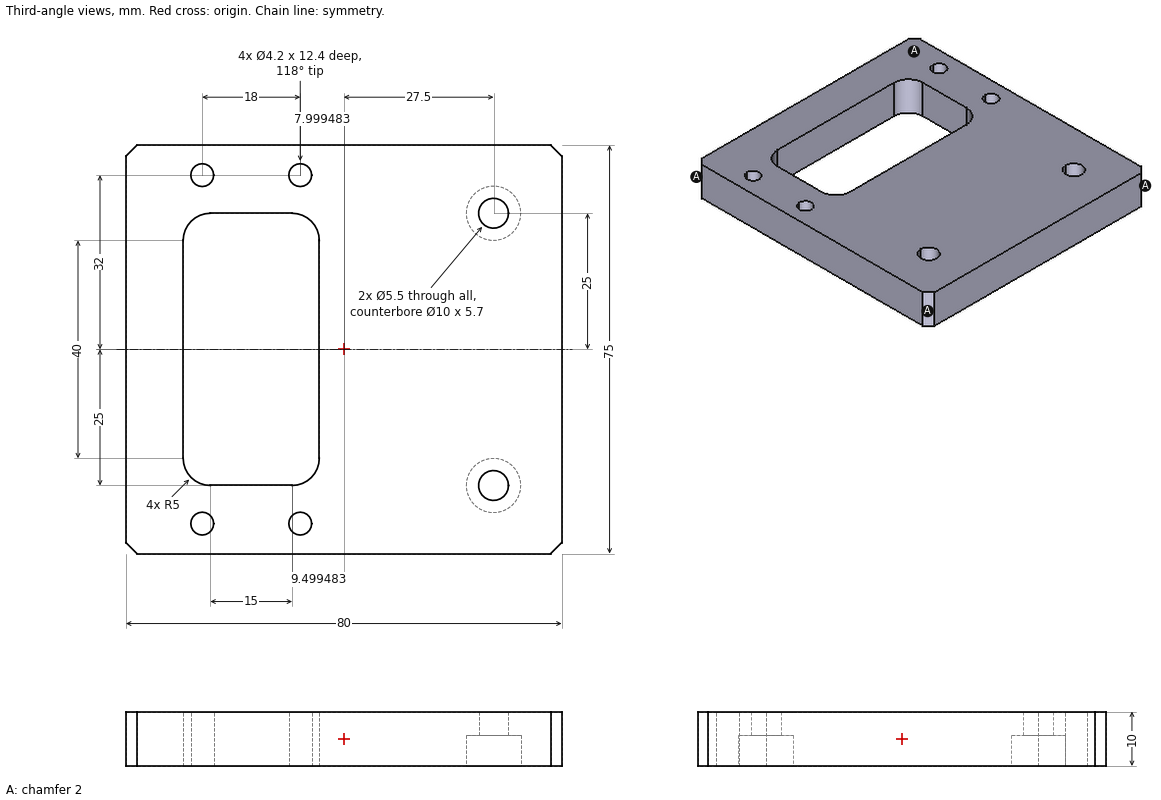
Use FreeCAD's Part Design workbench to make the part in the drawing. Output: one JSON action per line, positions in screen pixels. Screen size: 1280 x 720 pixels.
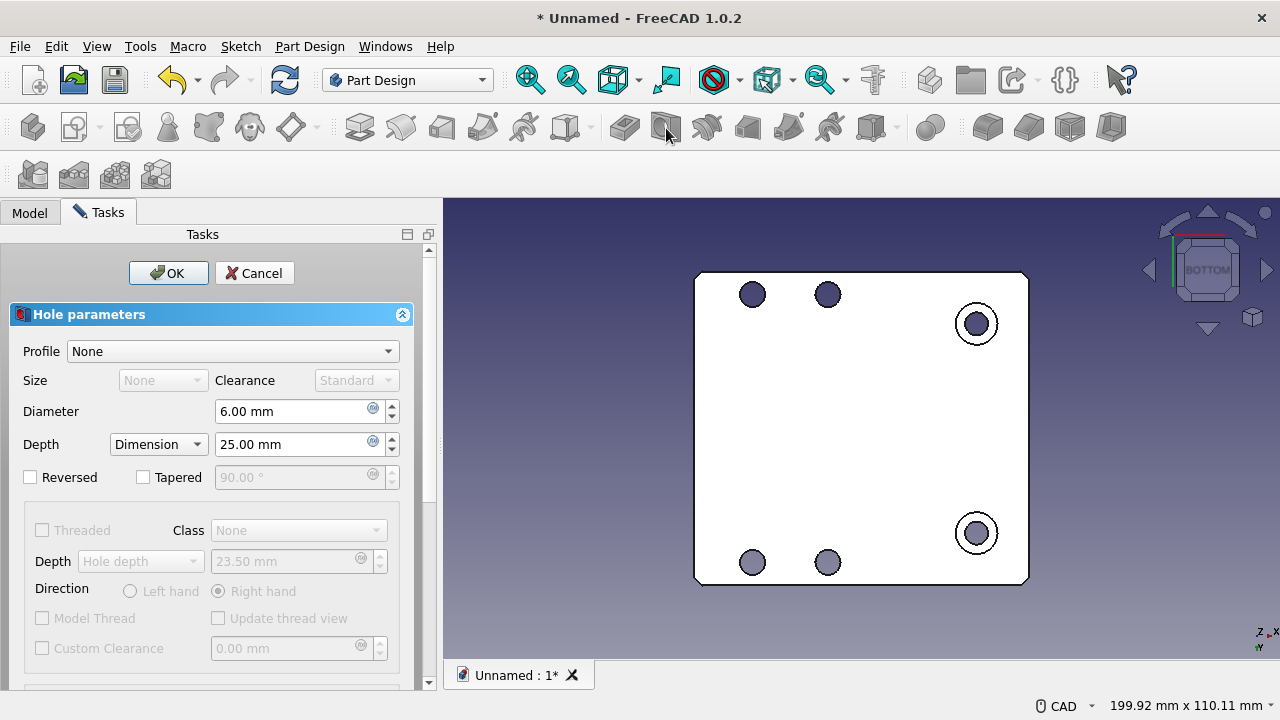
{"action": "triple_click", "coordinate": [300, 412]}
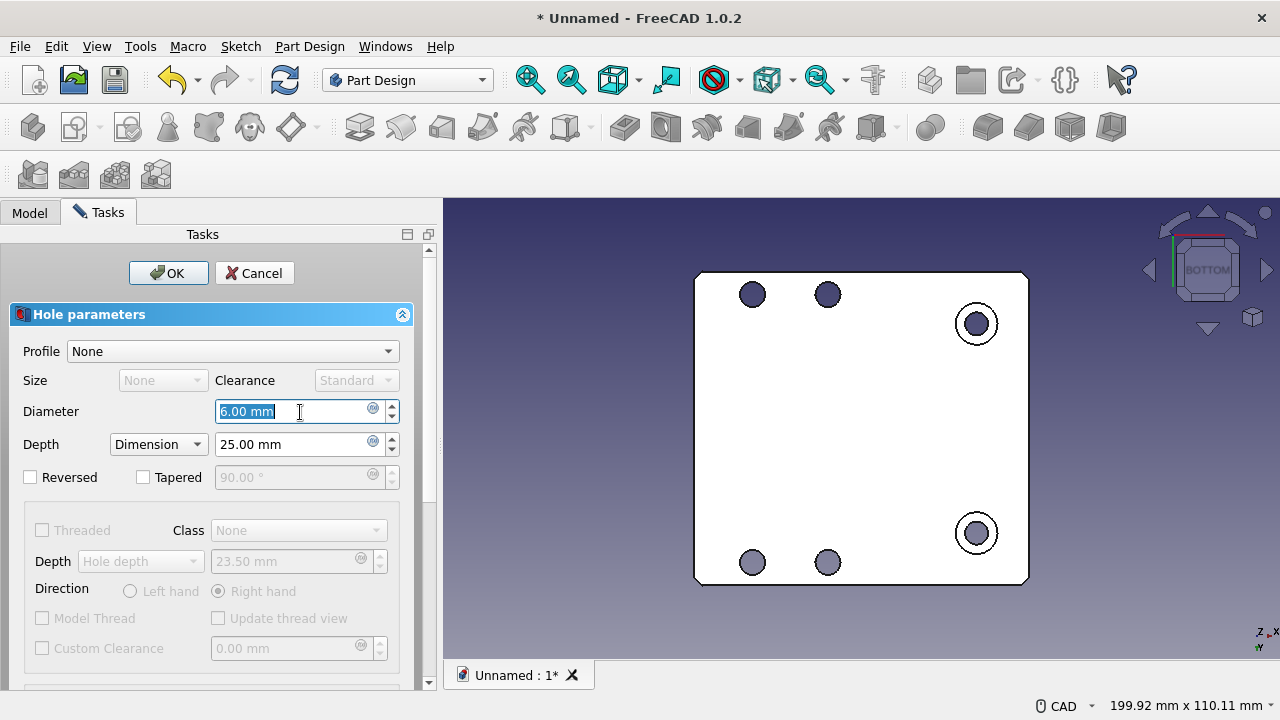
{"action": "type", "text": "4.2"}
{"action": "key", "text": "Tab"}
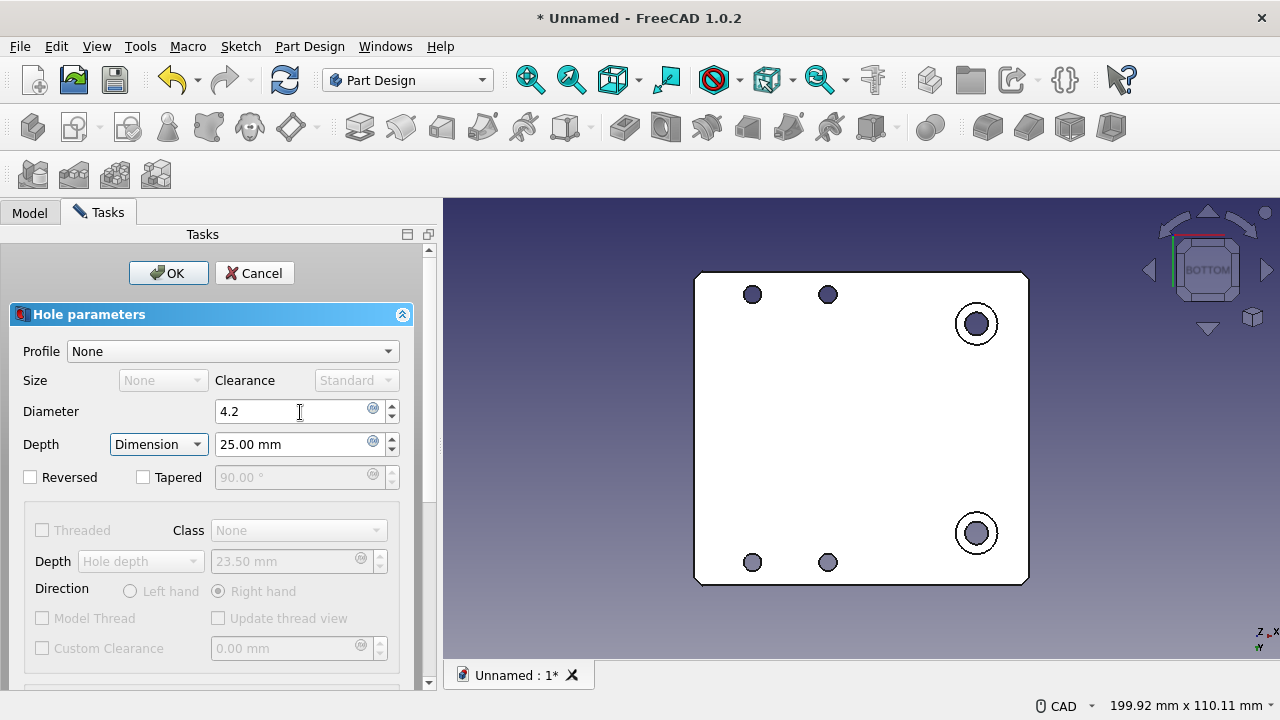
{"action": "triple_click", "coordinate": [300, 444]}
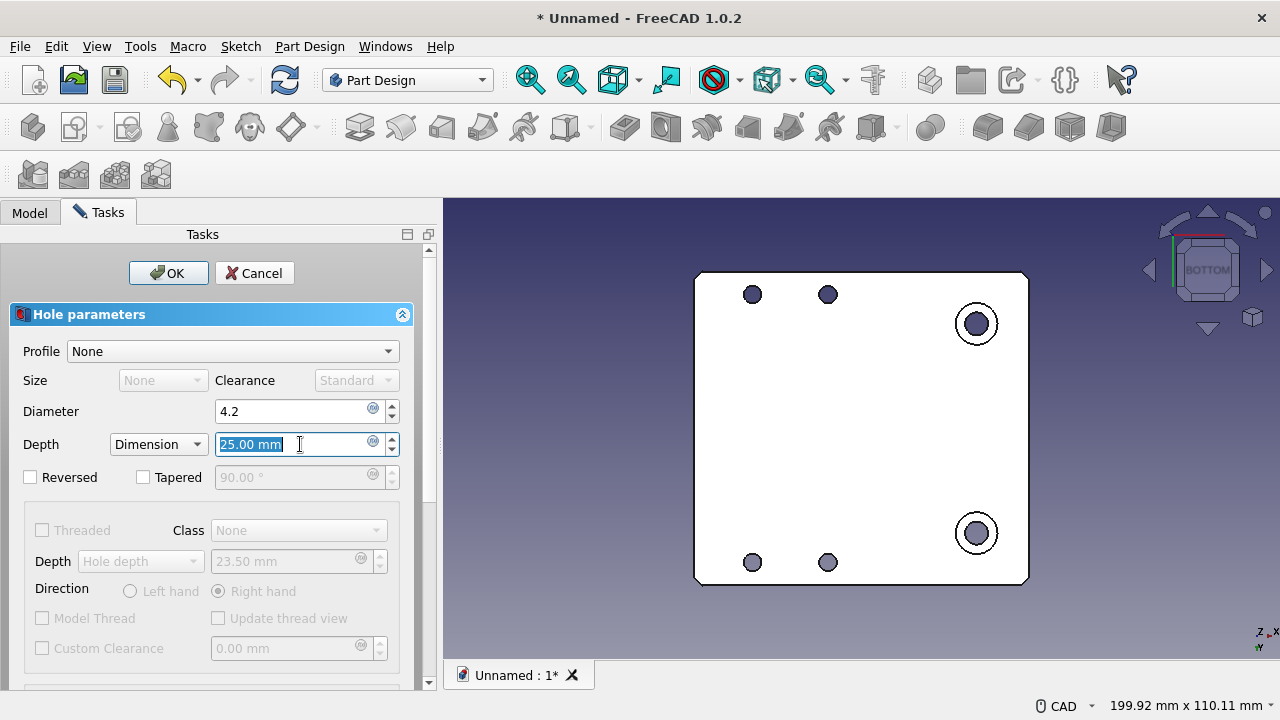
{"action": "type", "text": "12.4"}
{"action": "key", "text": "Tab"}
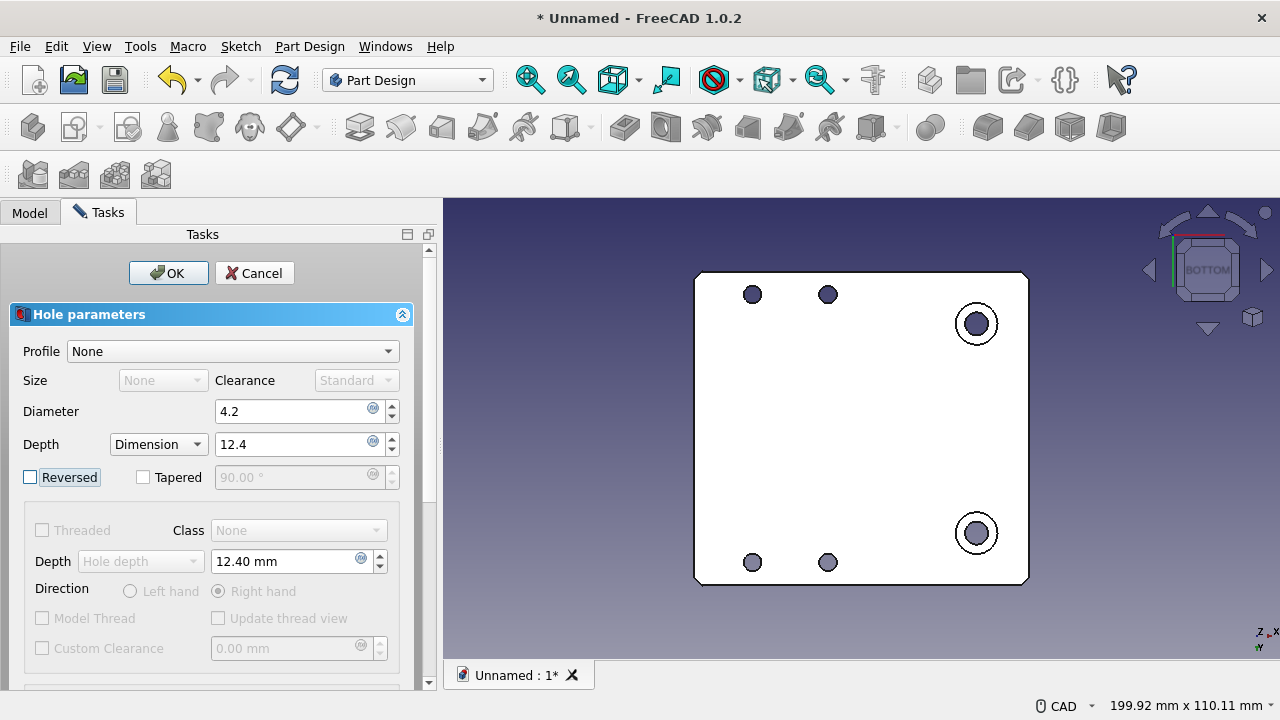
{"action": "left_click", "coordinate": [169, 273]}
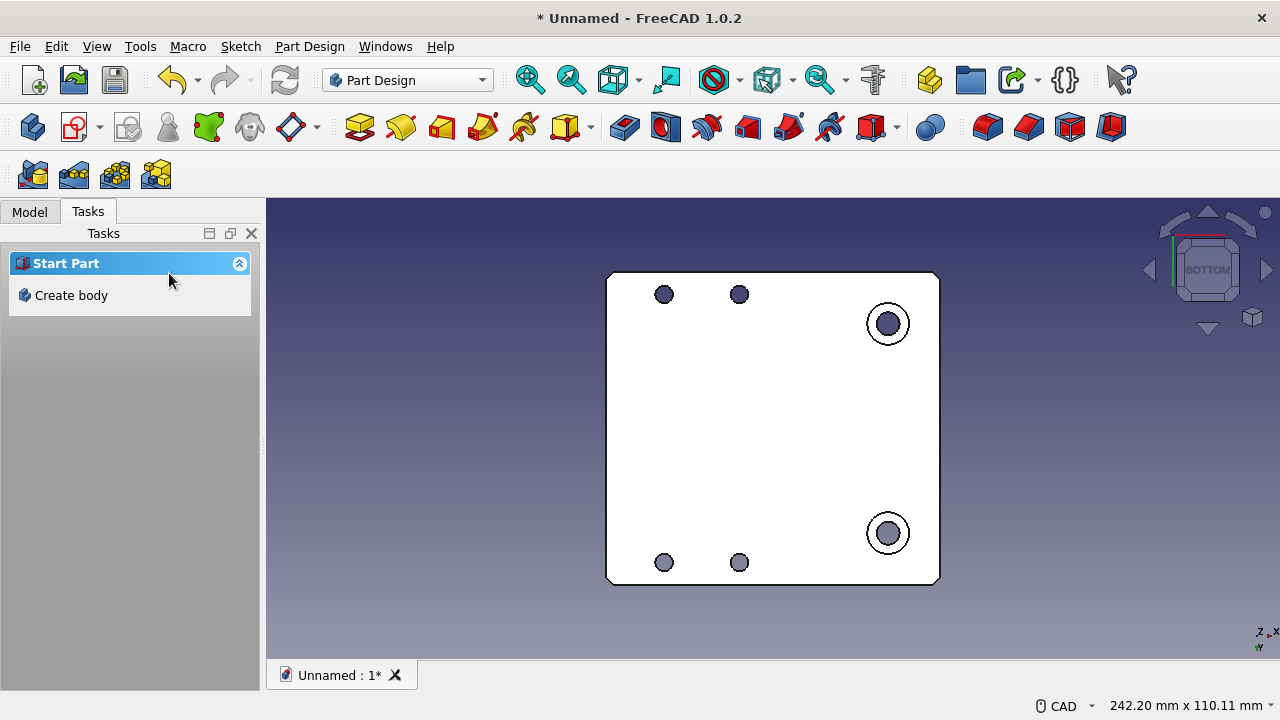
{"action": "left_click", "coordinate": [773, 428]}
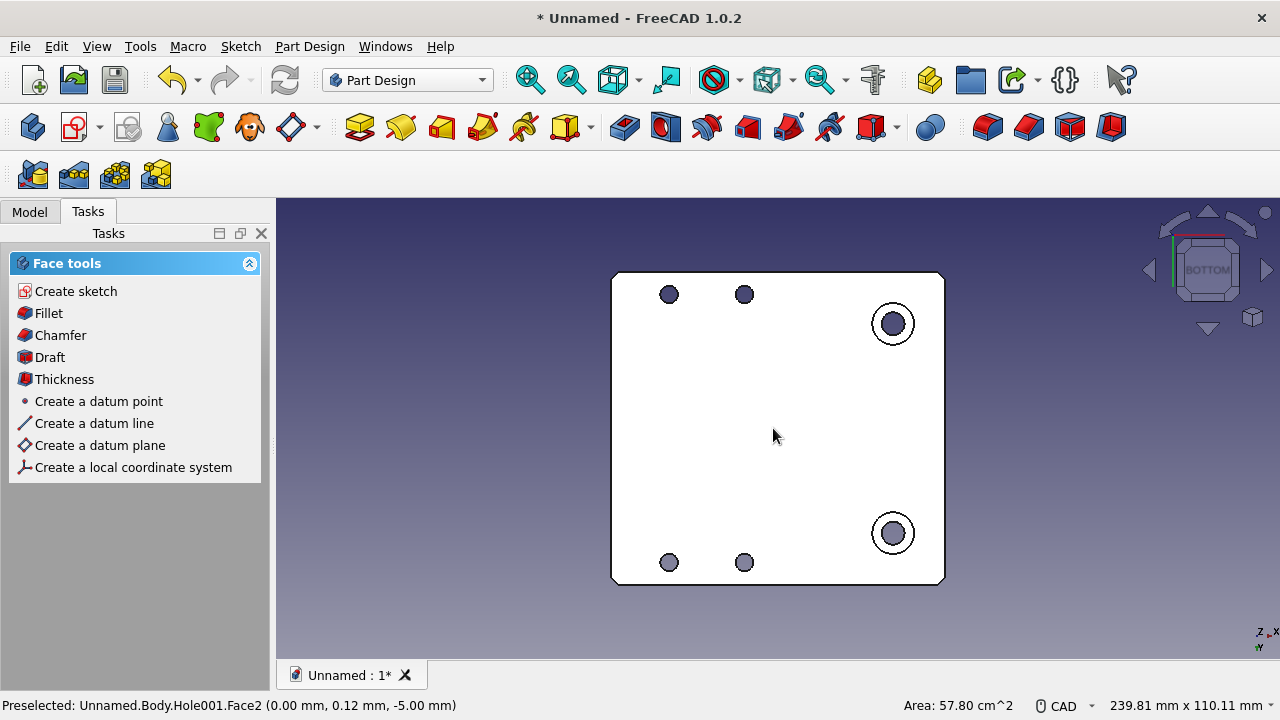
{"action": "left_click", "coordinate": [74, 128]}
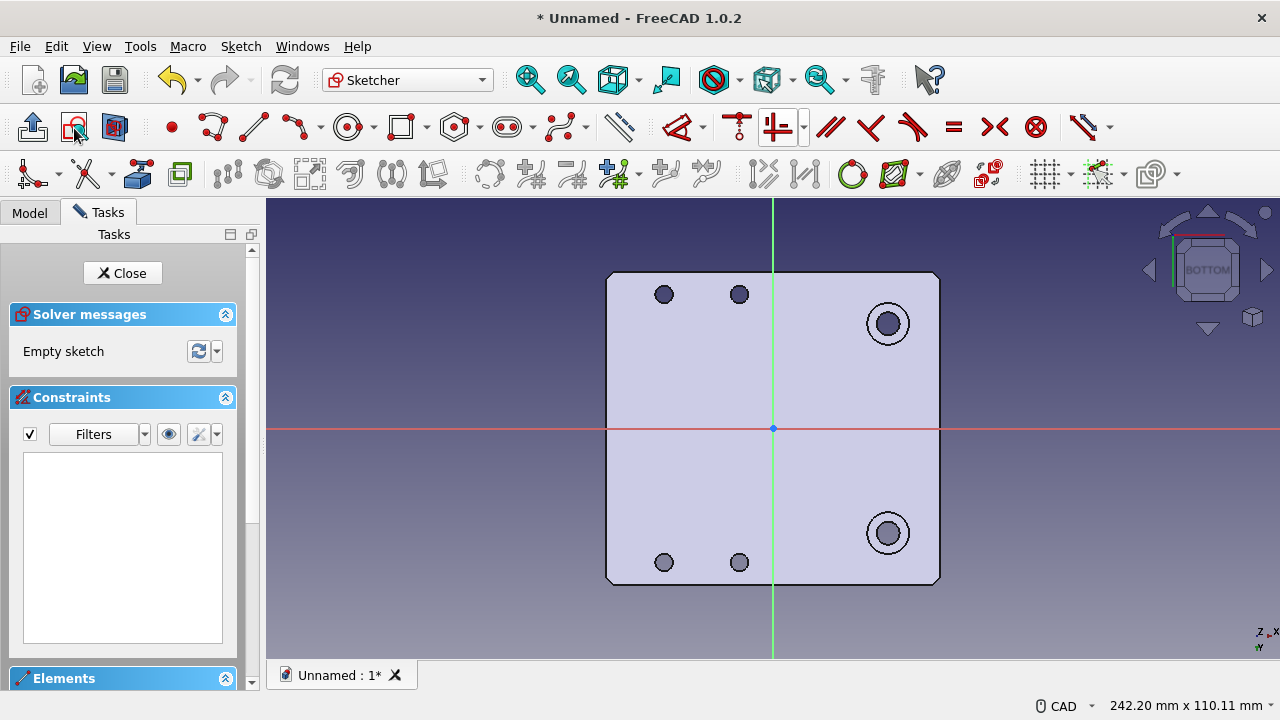
{"action": "scroll", "coordinate": [725, 429], "scroll_direction": "up", "scroll_amount": 2}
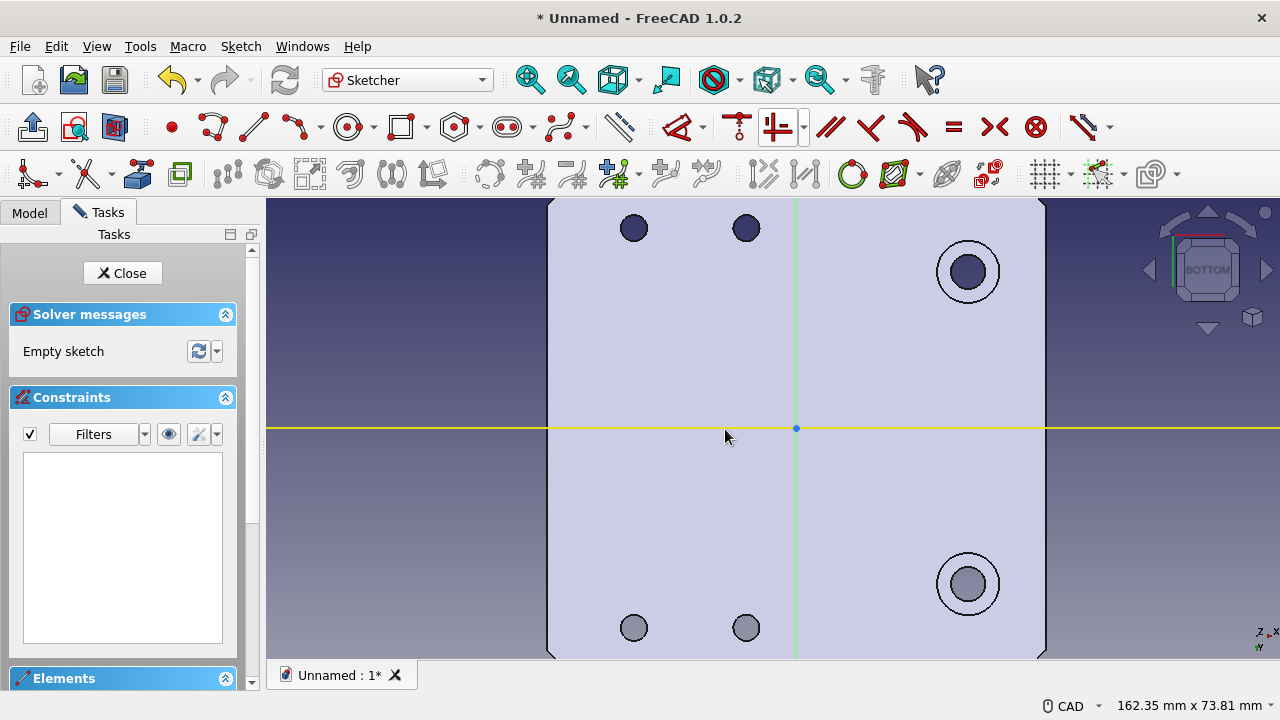
{"action": "key", "text": "g l"}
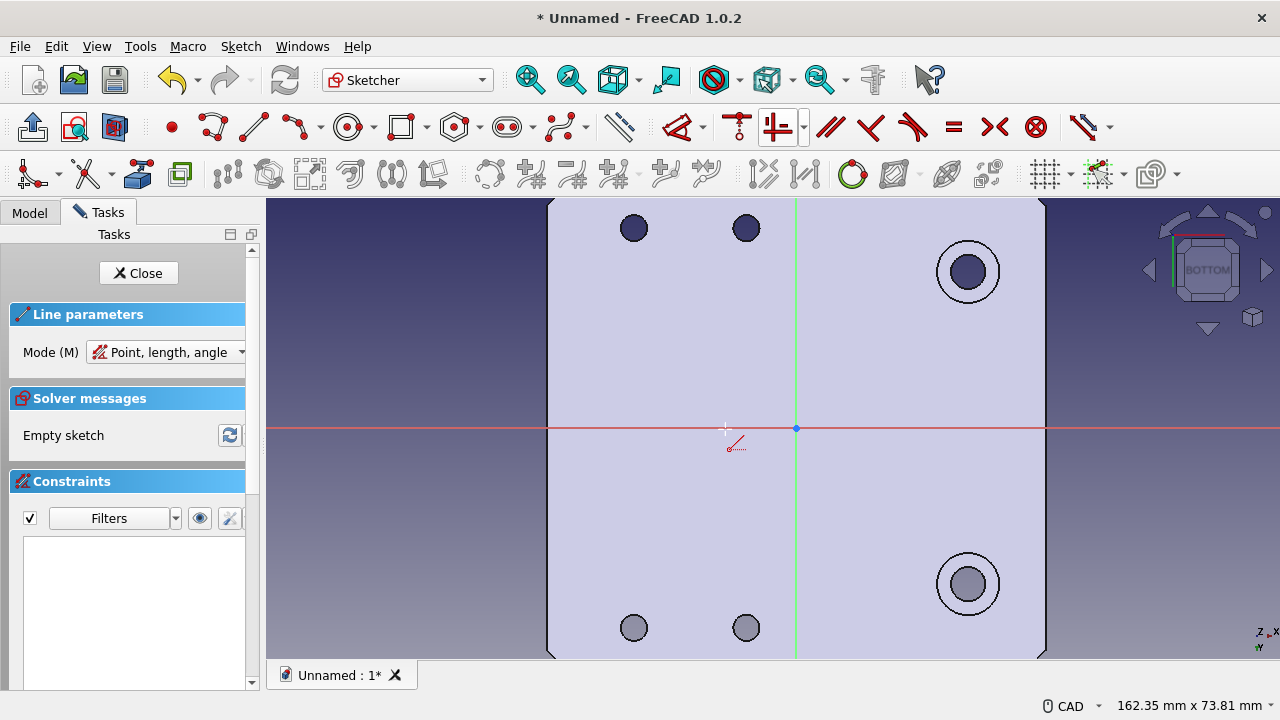
{"action": "left_click", "coordinate": [737, 272]}
{"action": "left_click", "coordinate": [643, 272]}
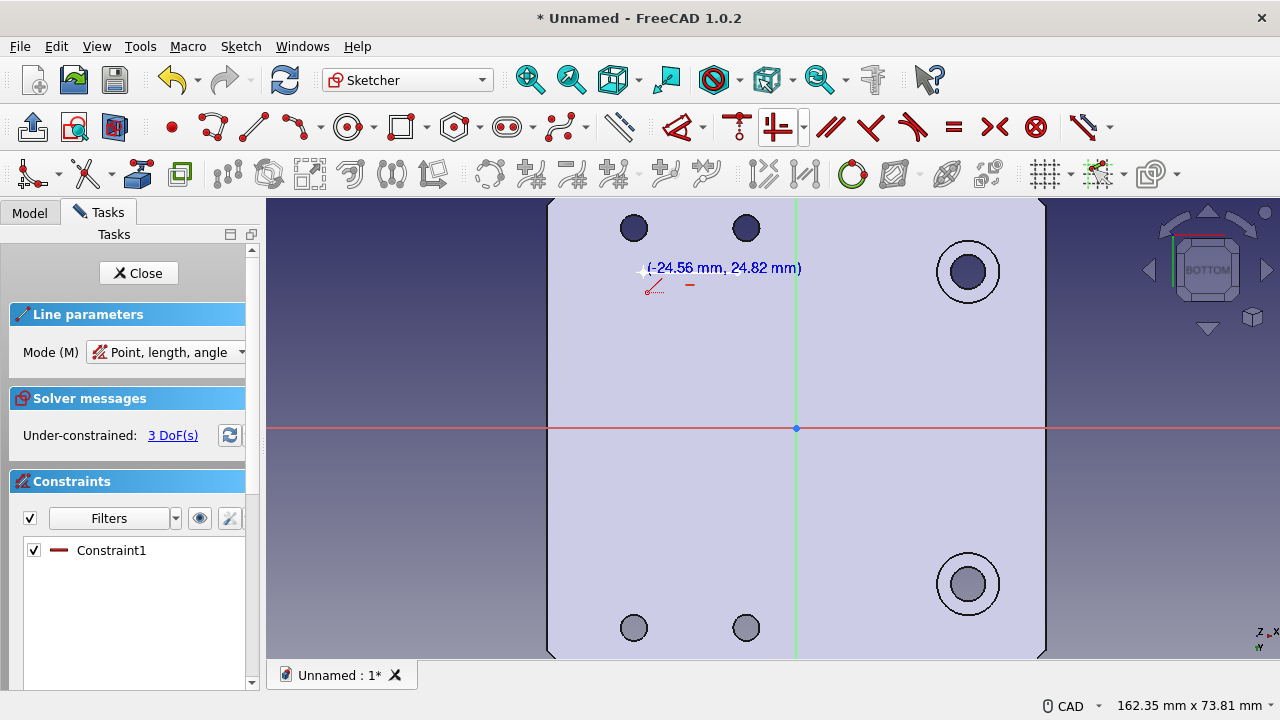
{"action": "left_click", "coordinate": [612, 303]}
{"action": "left_click", "coordinate": [612, 553]}